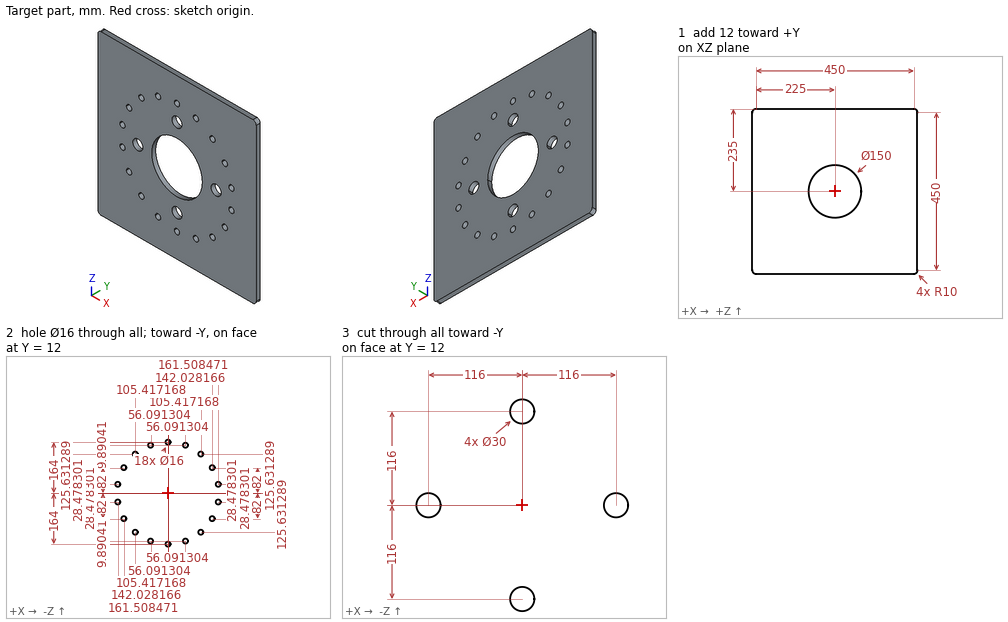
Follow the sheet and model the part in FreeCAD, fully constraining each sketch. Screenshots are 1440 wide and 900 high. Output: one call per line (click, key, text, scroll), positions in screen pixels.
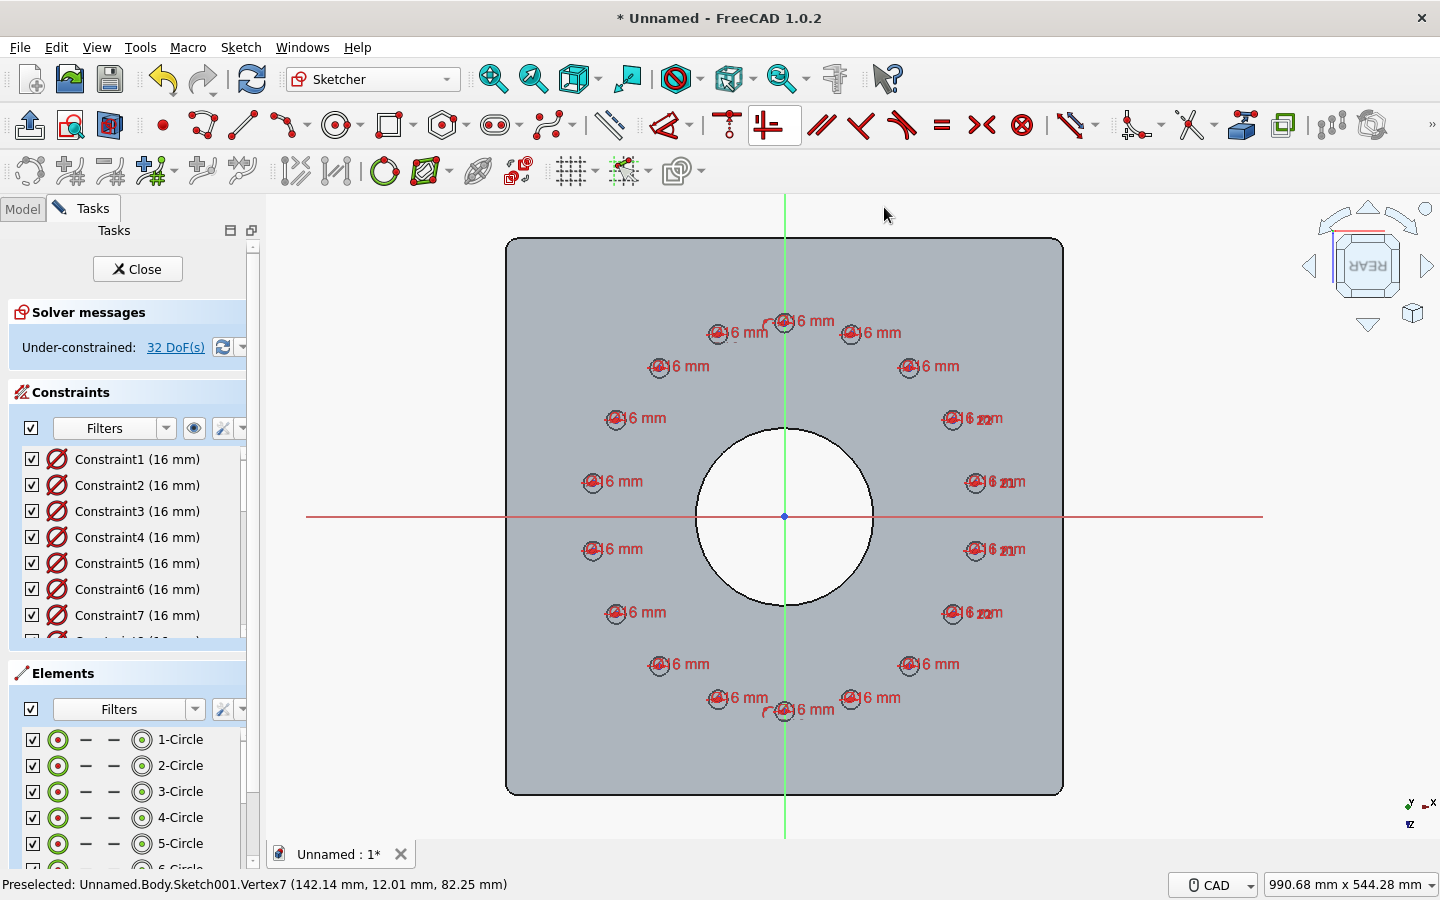
click(909, 368)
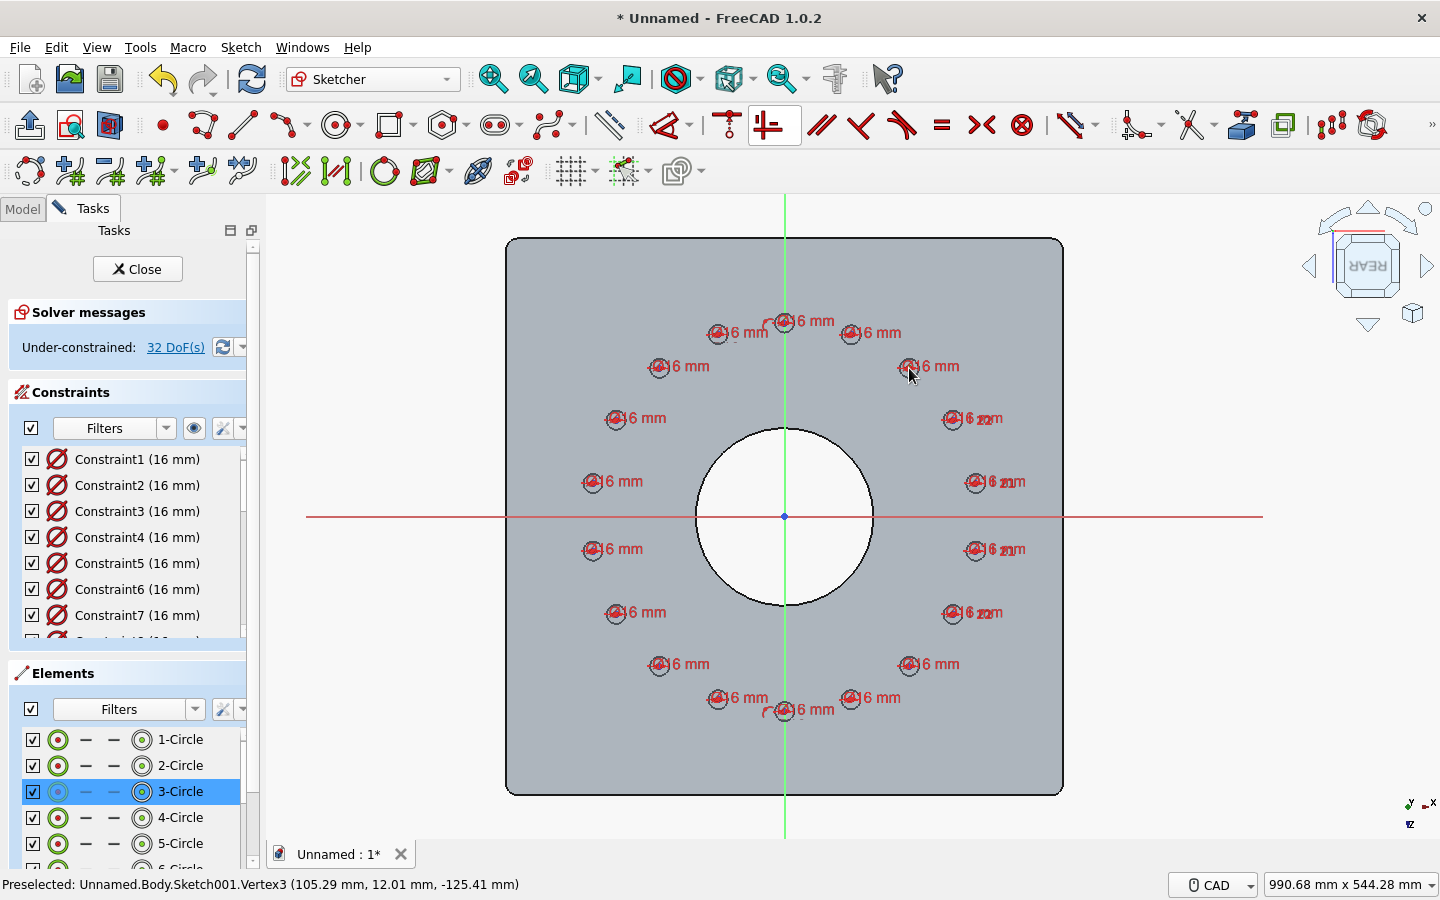
click(910, 666)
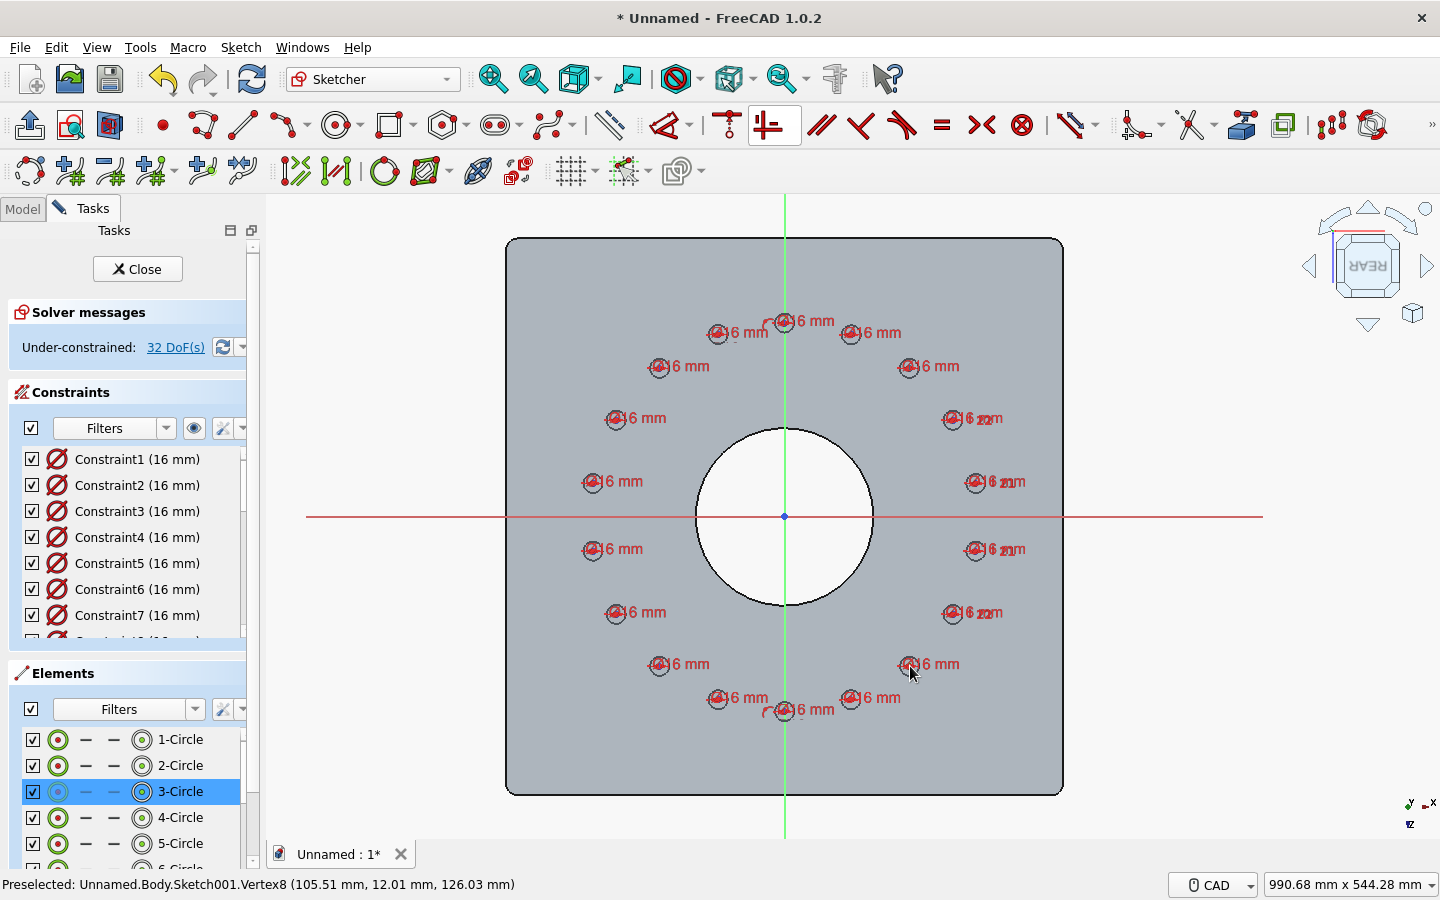
key(v)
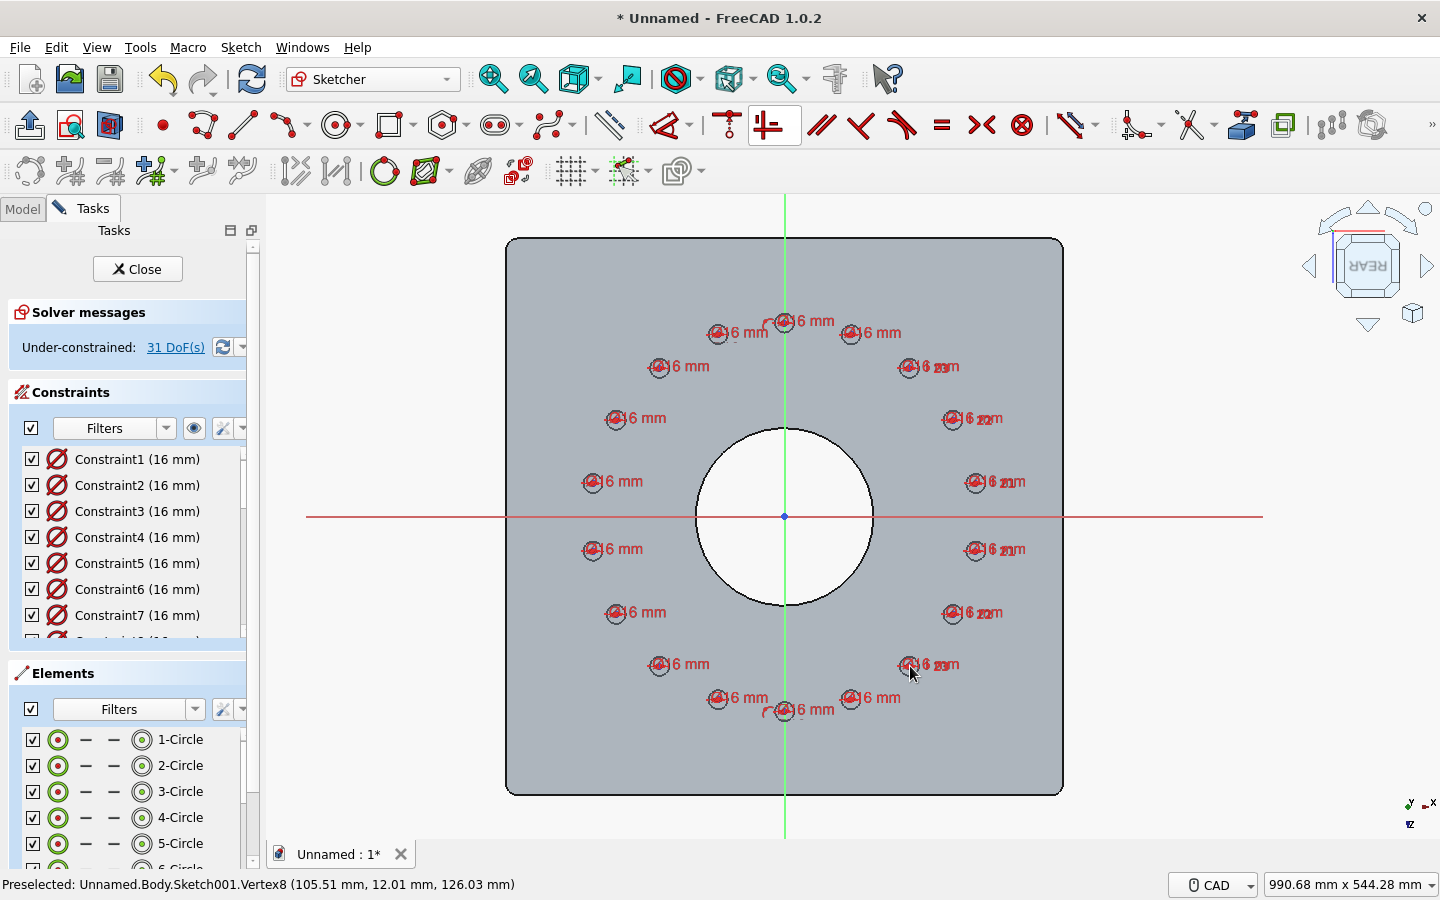
click(851, 700)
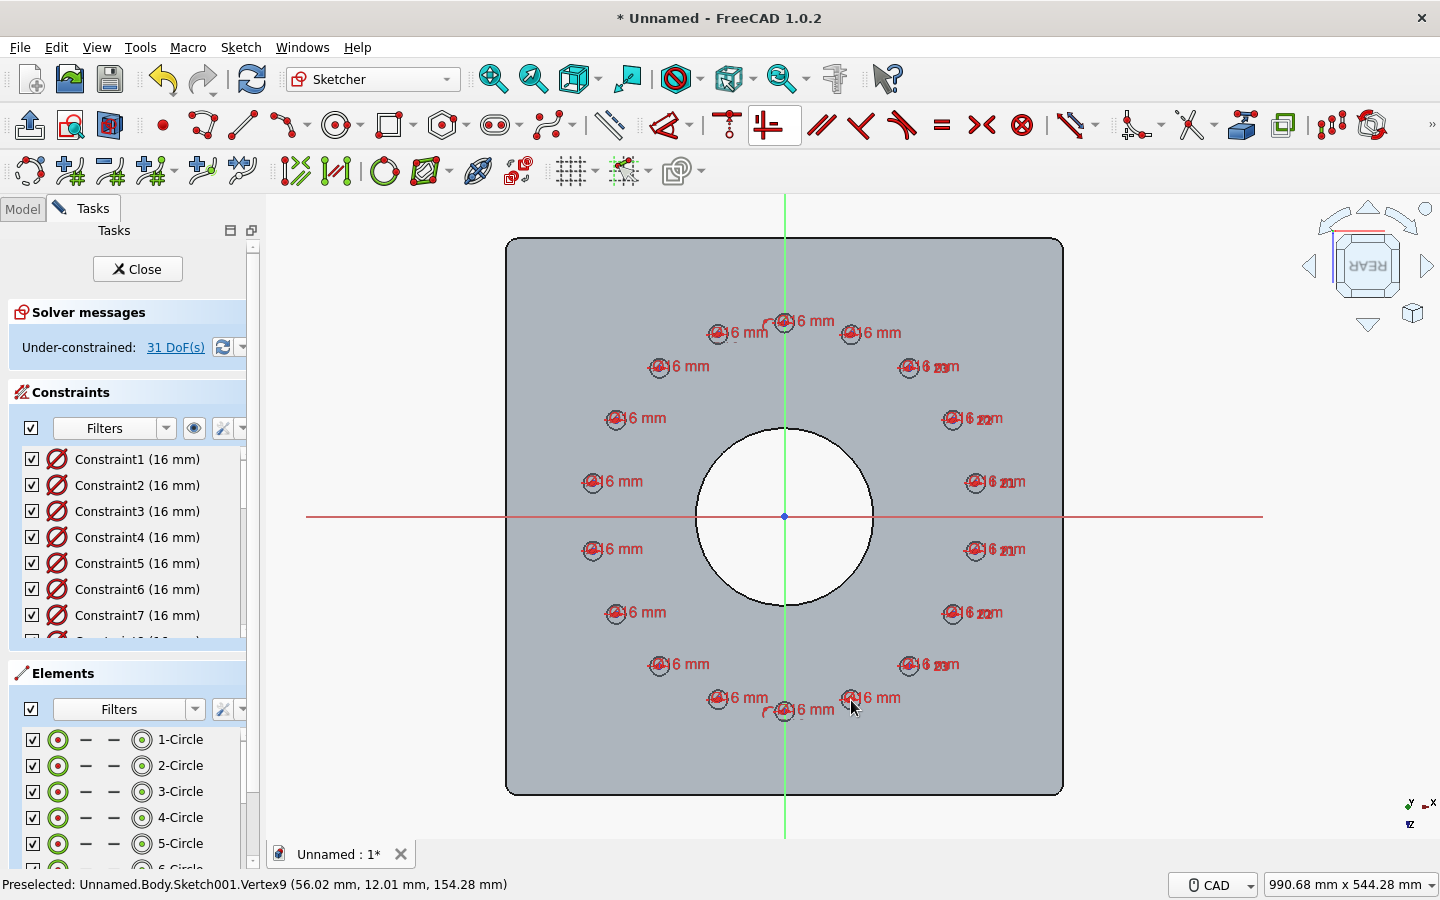
click(718, 700)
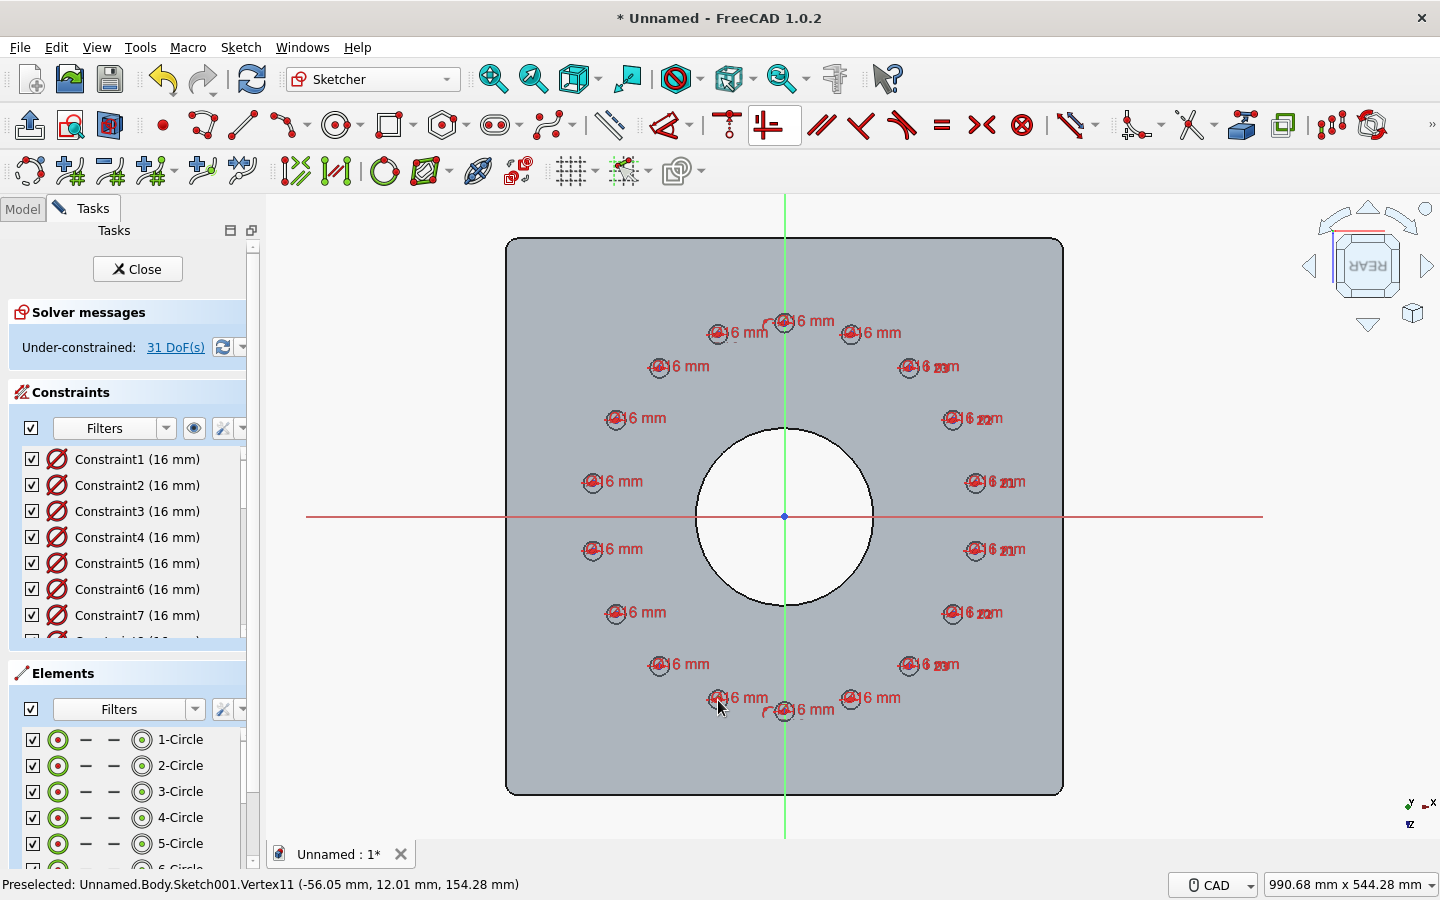
key(h)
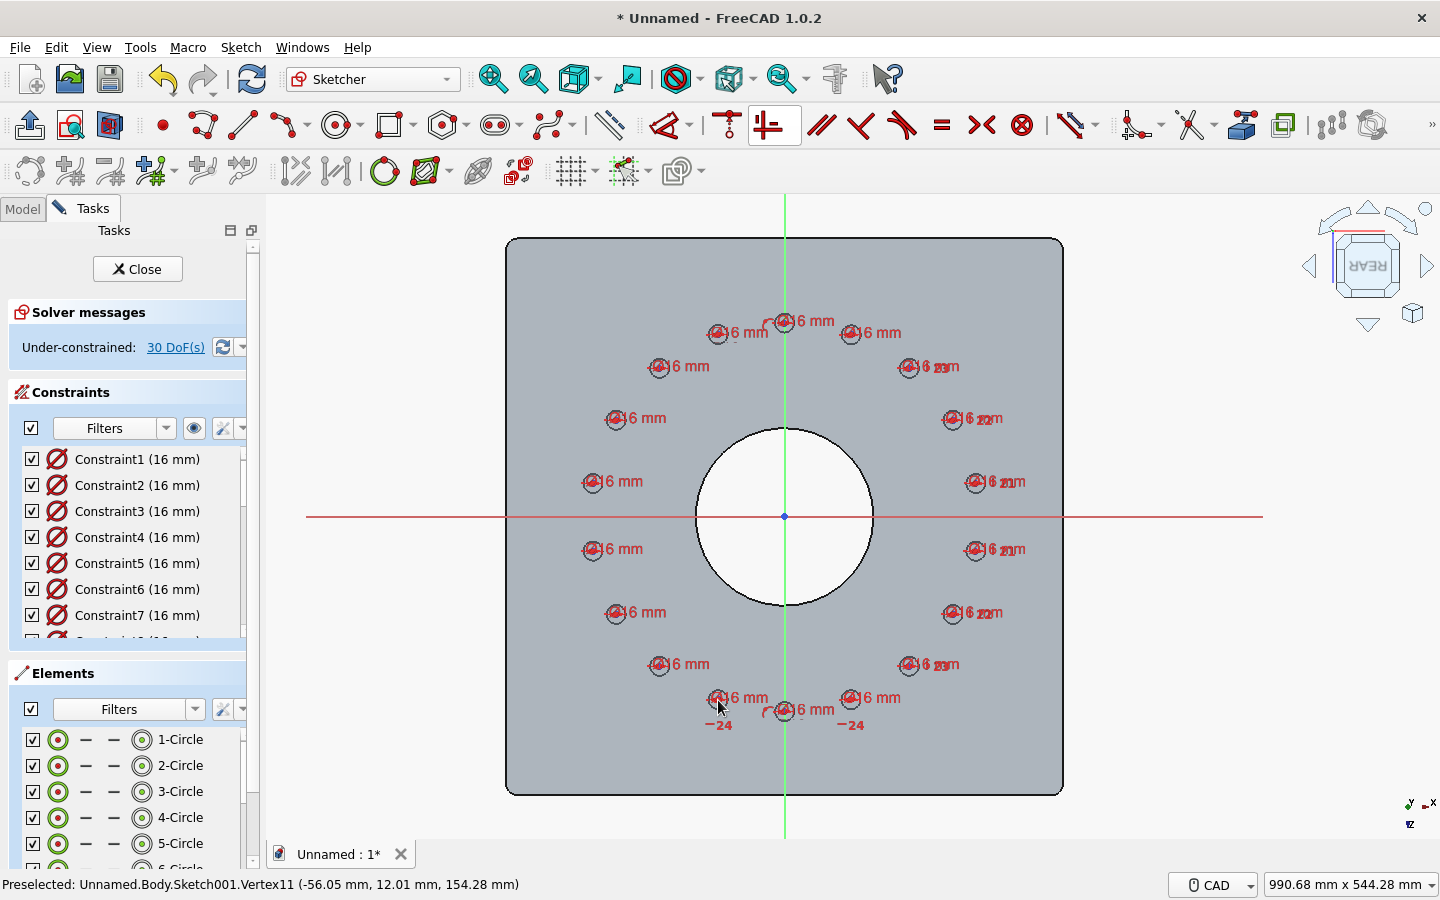
click(909, 666)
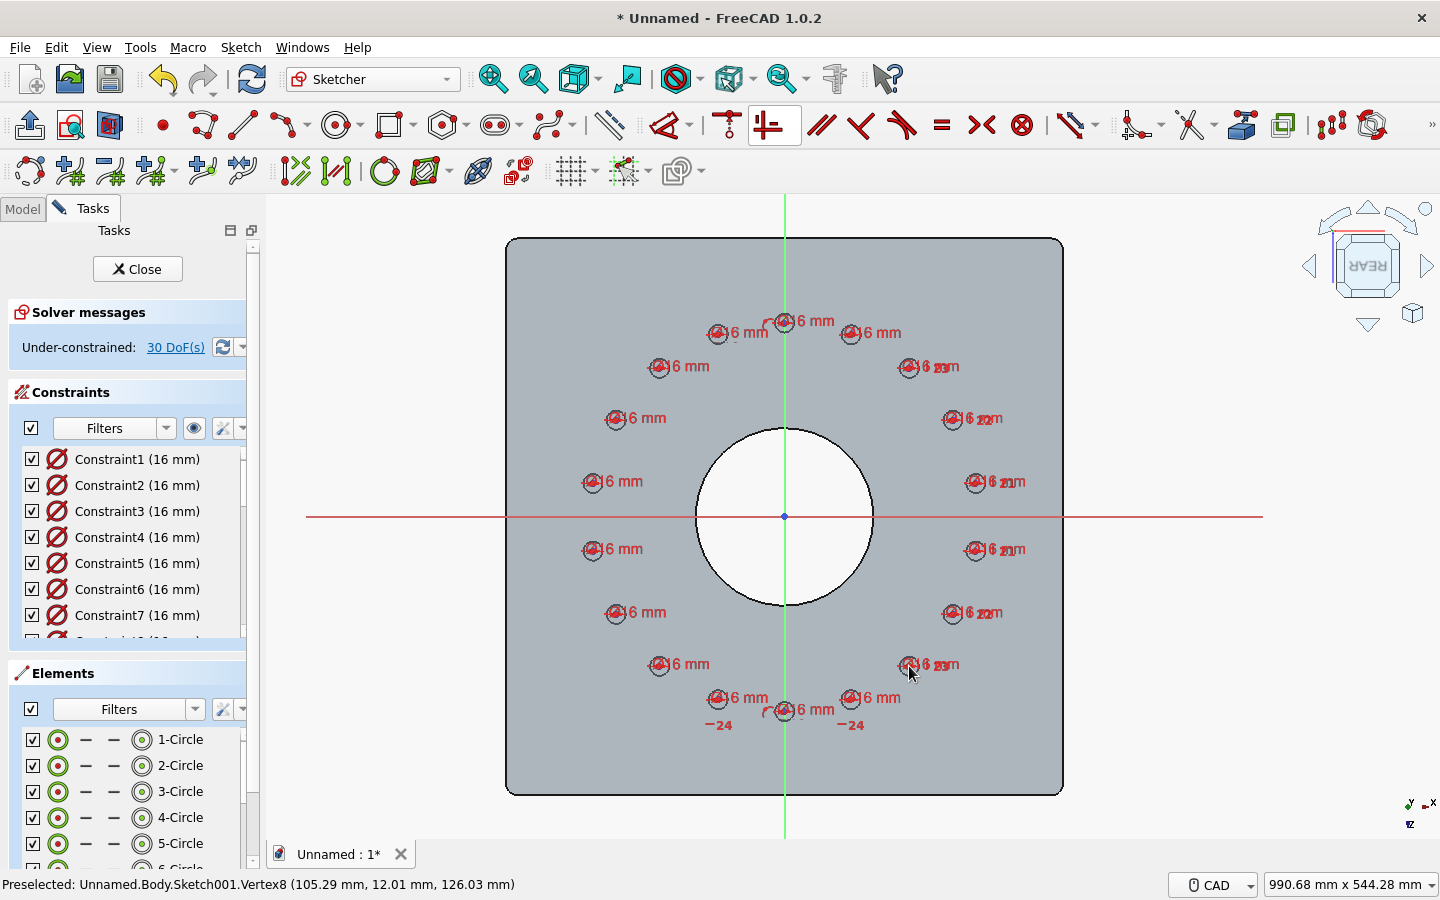
click(660, 666)